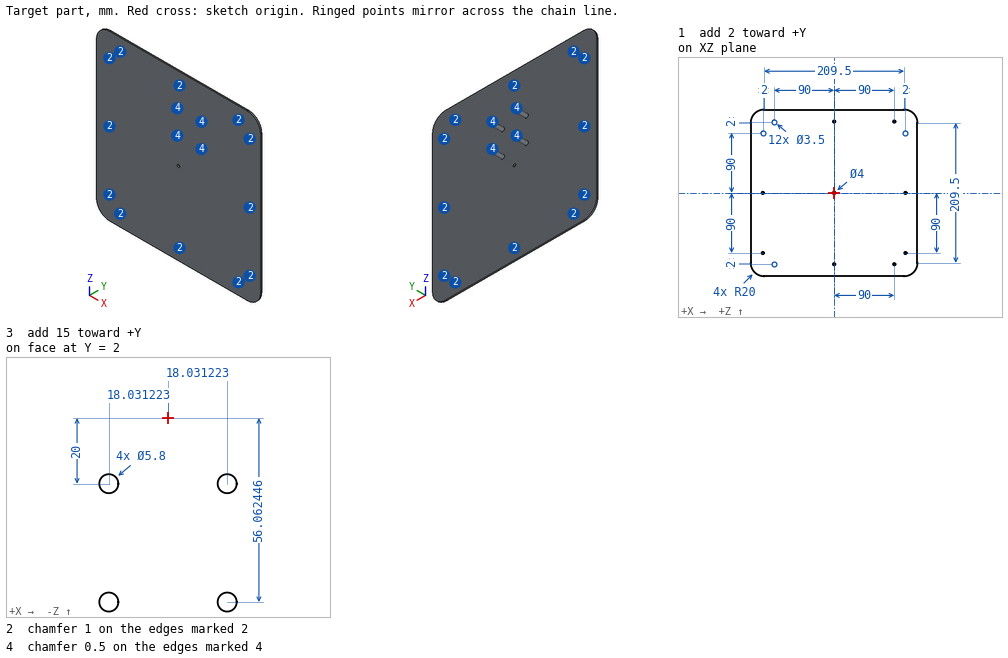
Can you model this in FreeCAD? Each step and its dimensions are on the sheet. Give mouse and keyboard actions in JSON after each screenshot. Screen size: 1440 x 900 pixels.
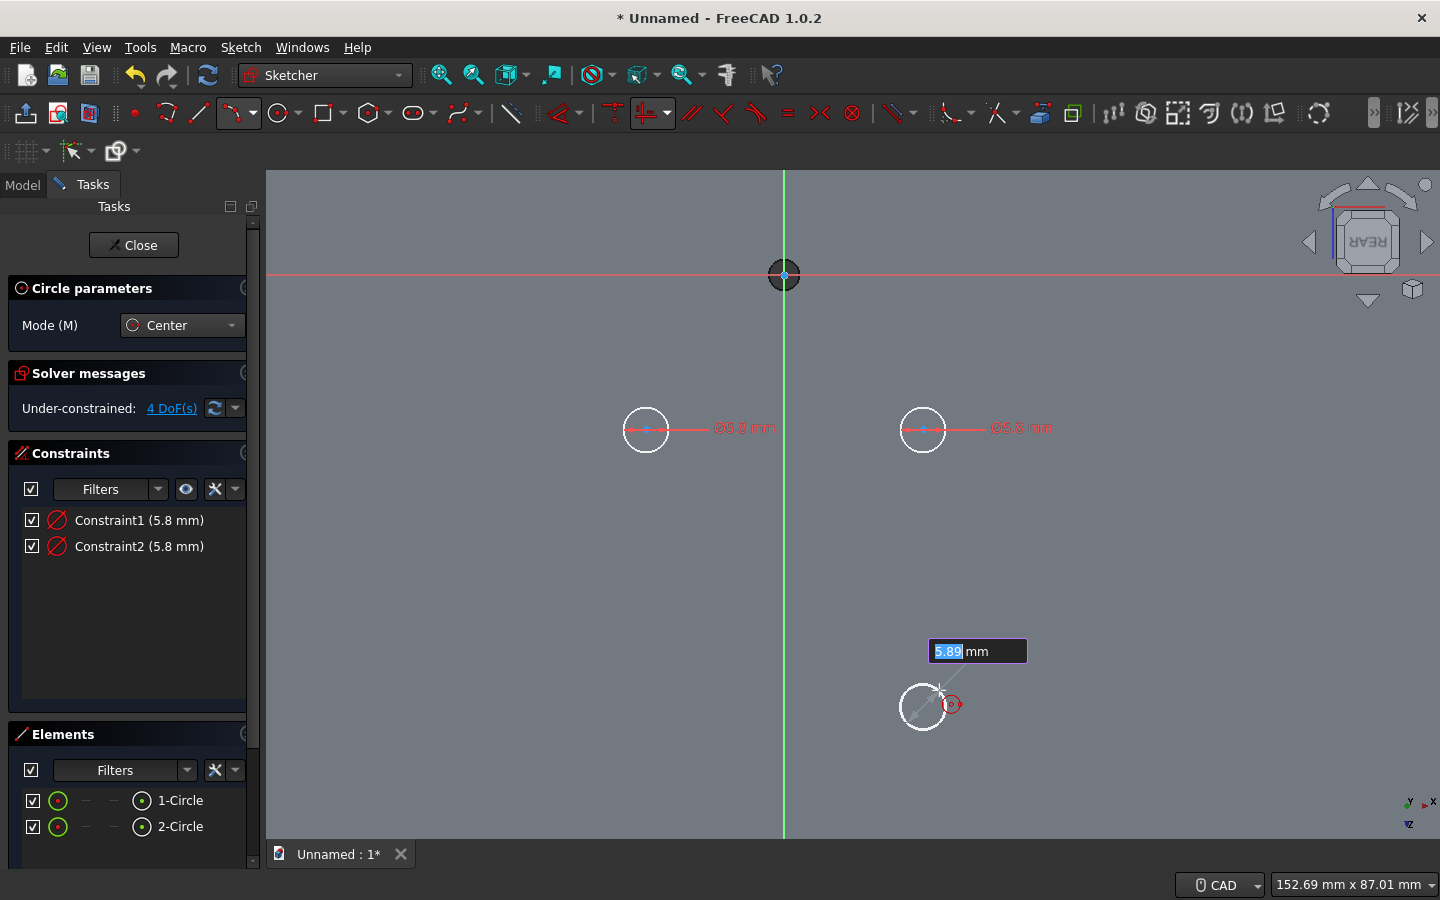
{"action": "type", "text": "5.8"}
{"action": "key", "text": "Return"}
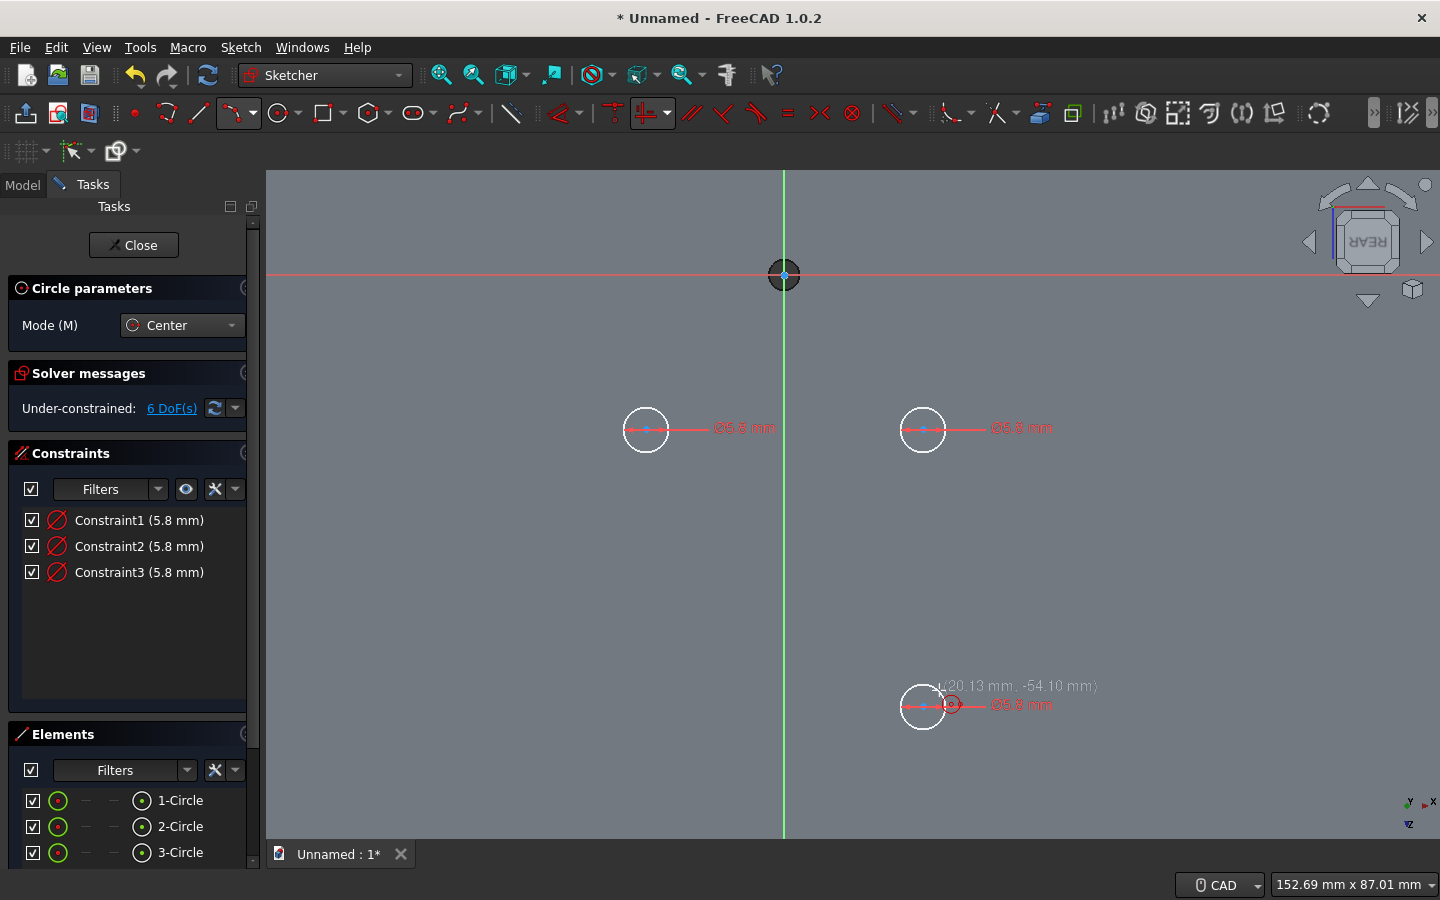
{"action": "left_click", "coordinate": [646, 706]}
{"action": "mouse_move", "coordinate": [661, 690]}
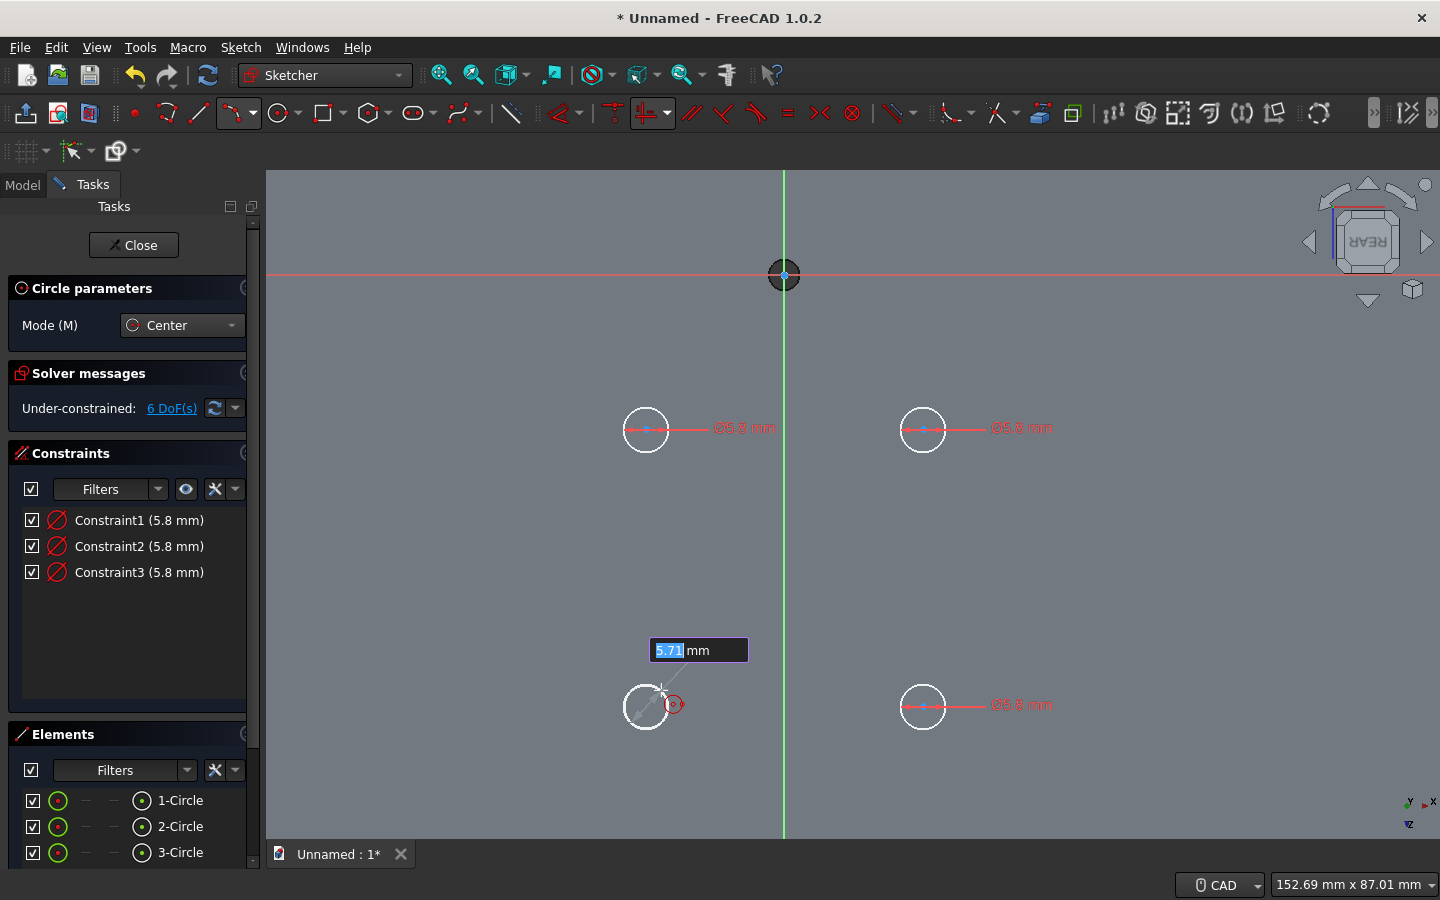
{"action": "type", "text": "5.8"}
{"action": "key", "text": "Return"}
{"action": "key", "text": "Escape"}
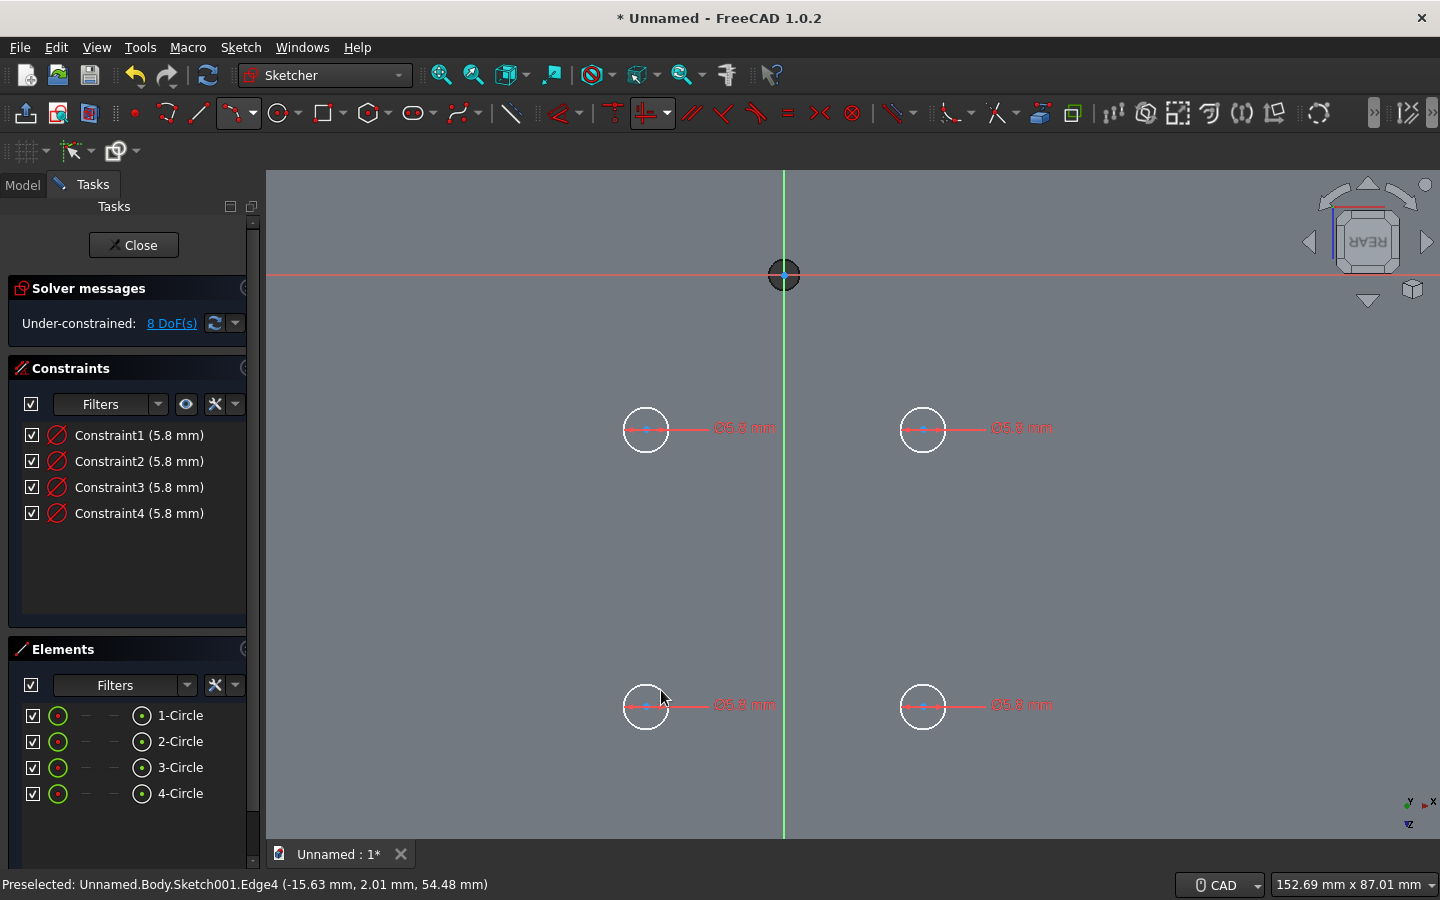
{"action": "left_click", "coordinate": [646, 430]}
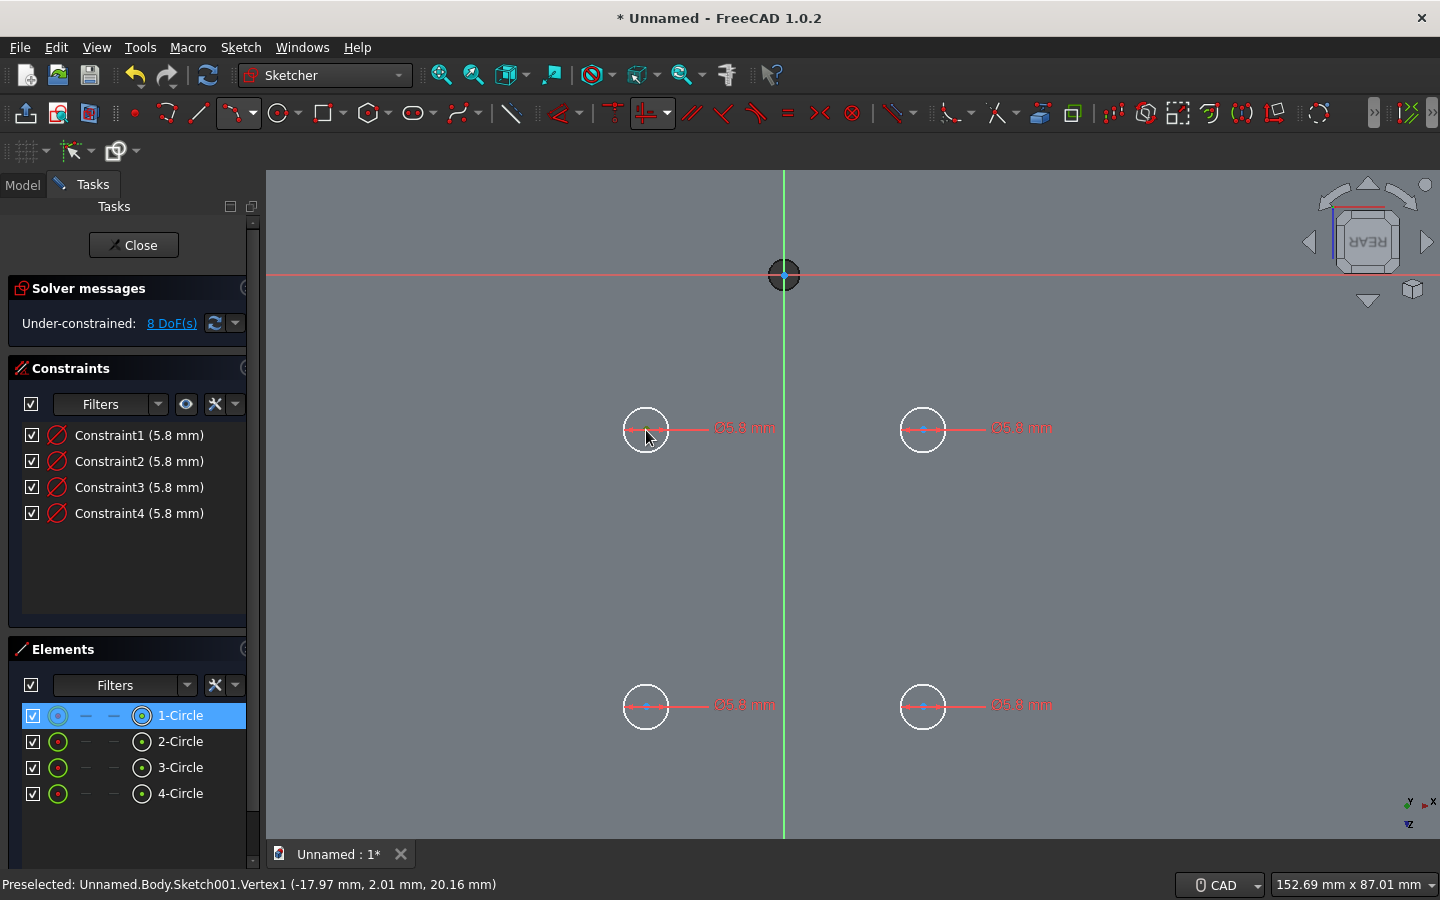
{"action": "left_click", "coordinate": [923, 430]}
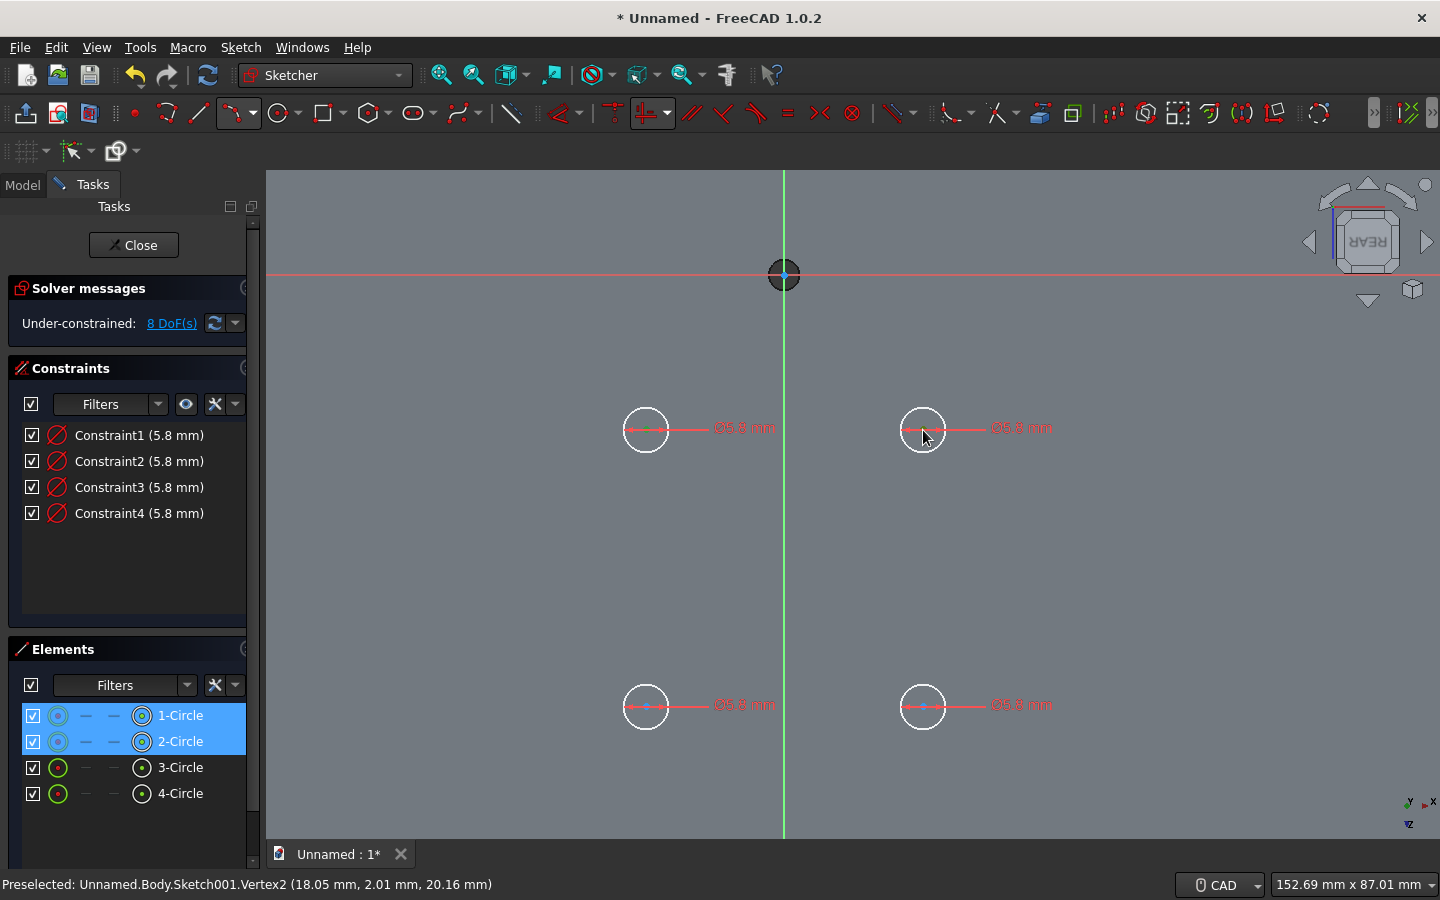
{"action": "key", "text": "h"}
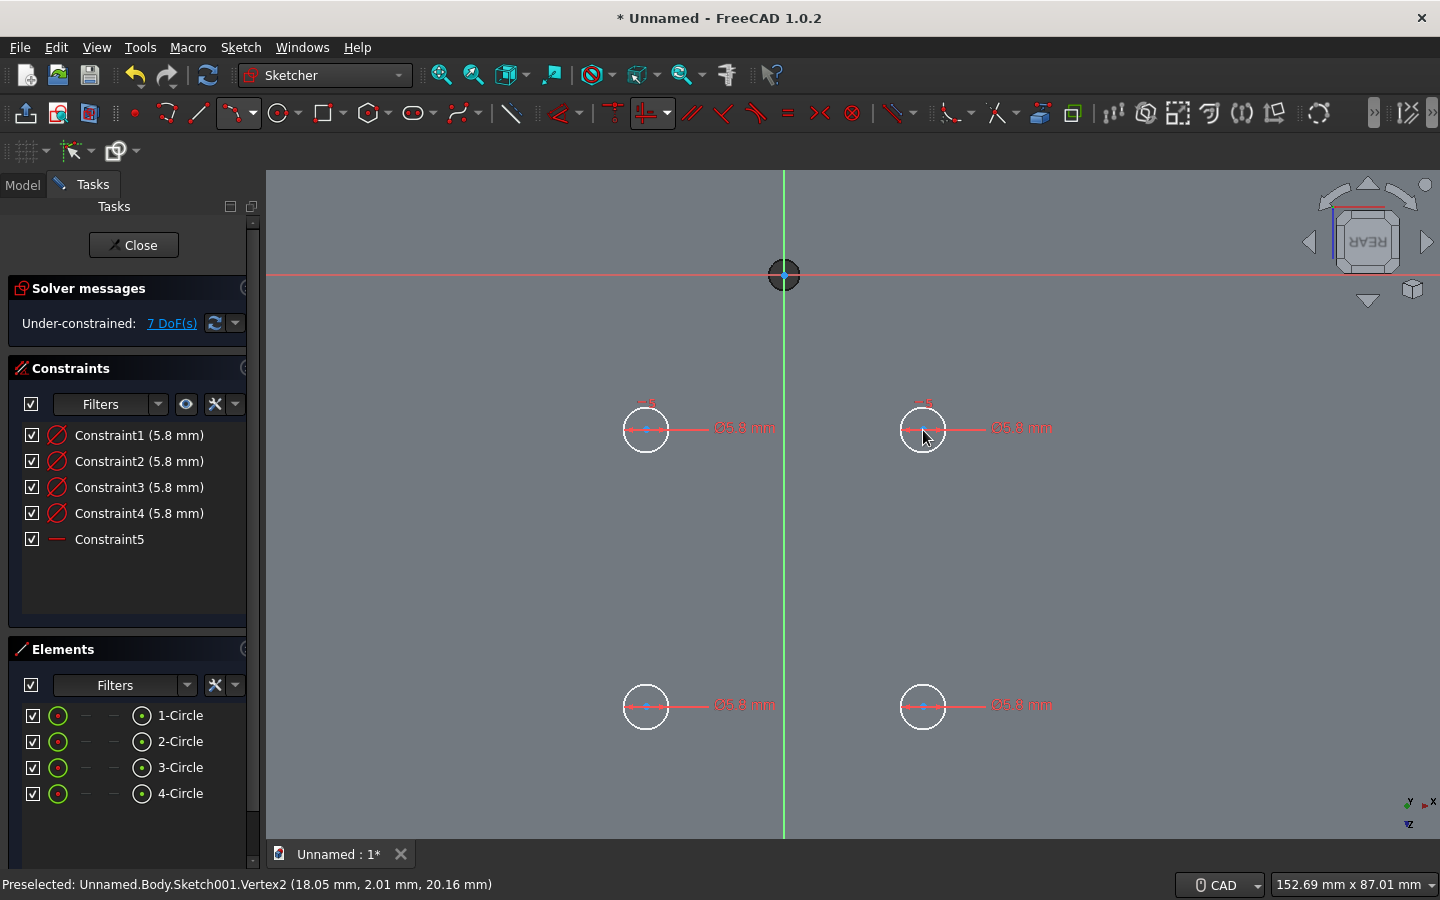
{"action": "left_click", "coordinate": [923, 430]}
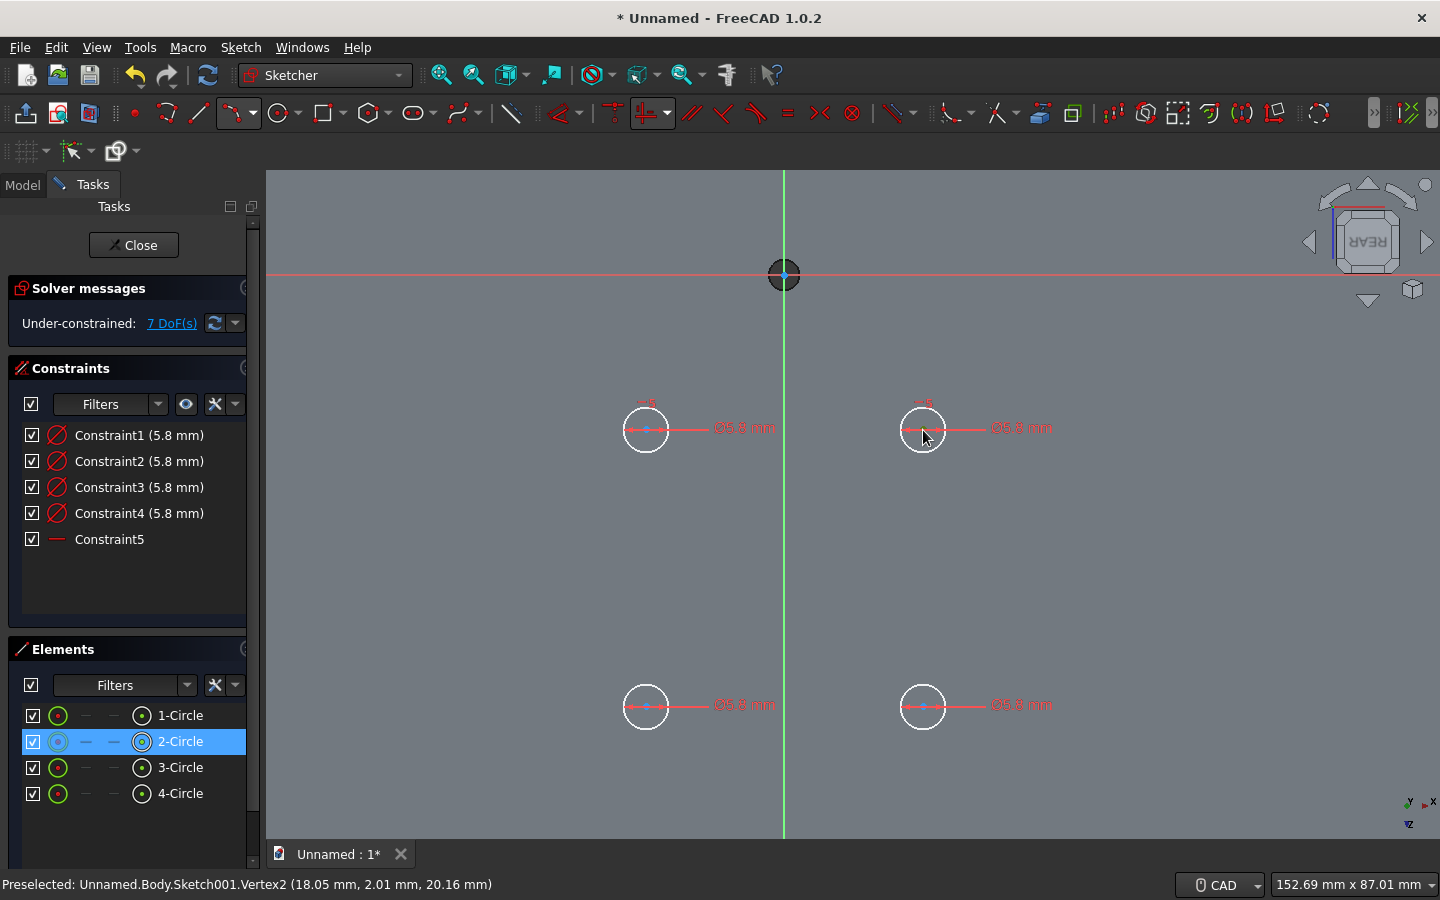
{"action": "left_click", "coordinate": [923, 707]}